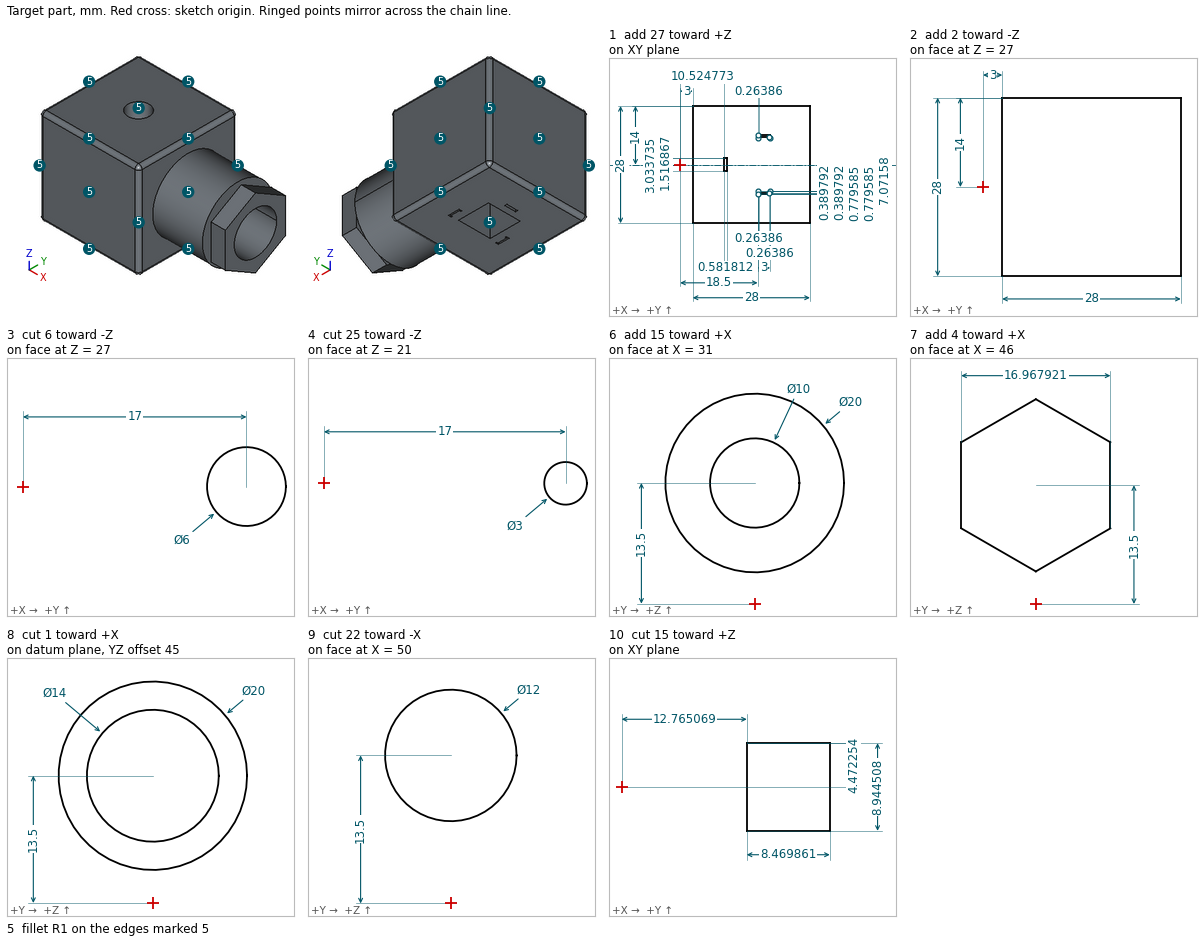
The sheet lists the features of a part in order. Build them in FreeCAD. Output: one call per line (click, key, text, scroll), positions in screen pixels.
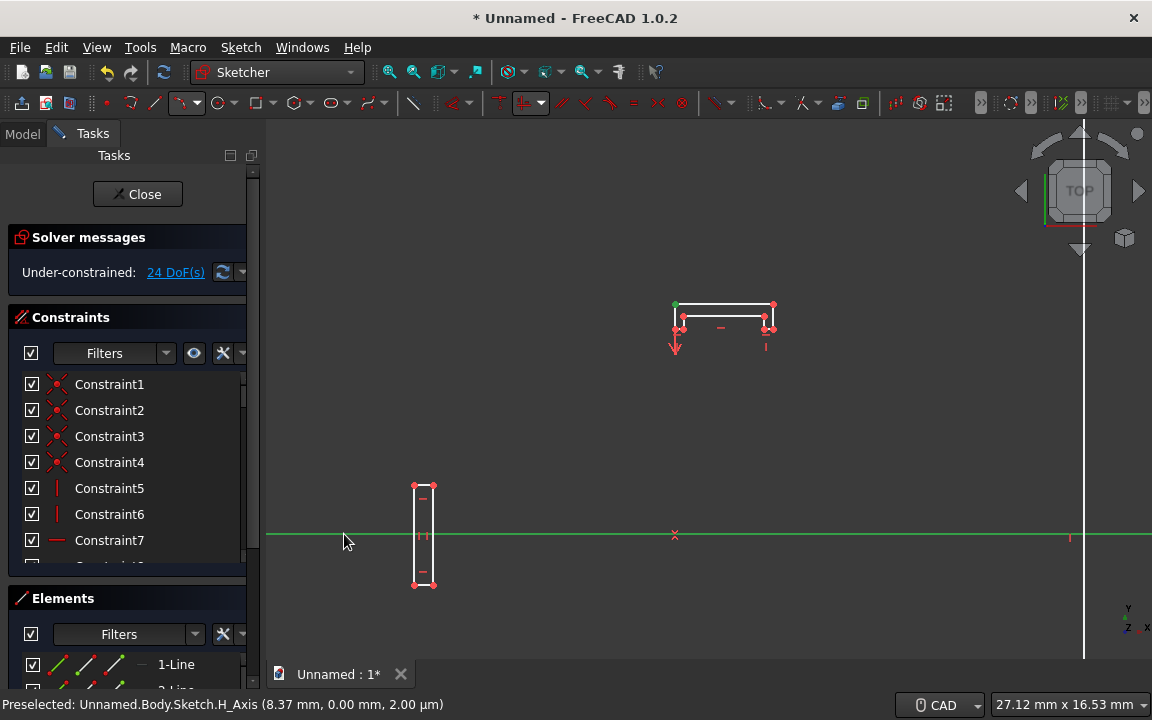
click(658, 104)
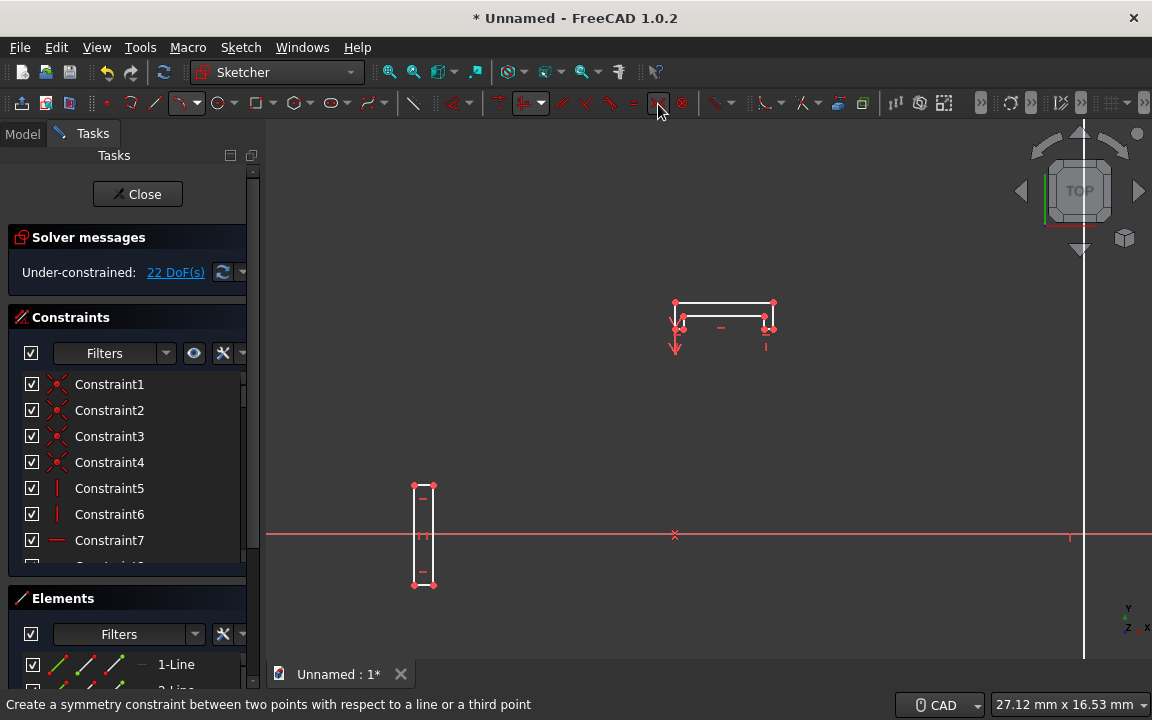
scroll(677, 304, down, 5)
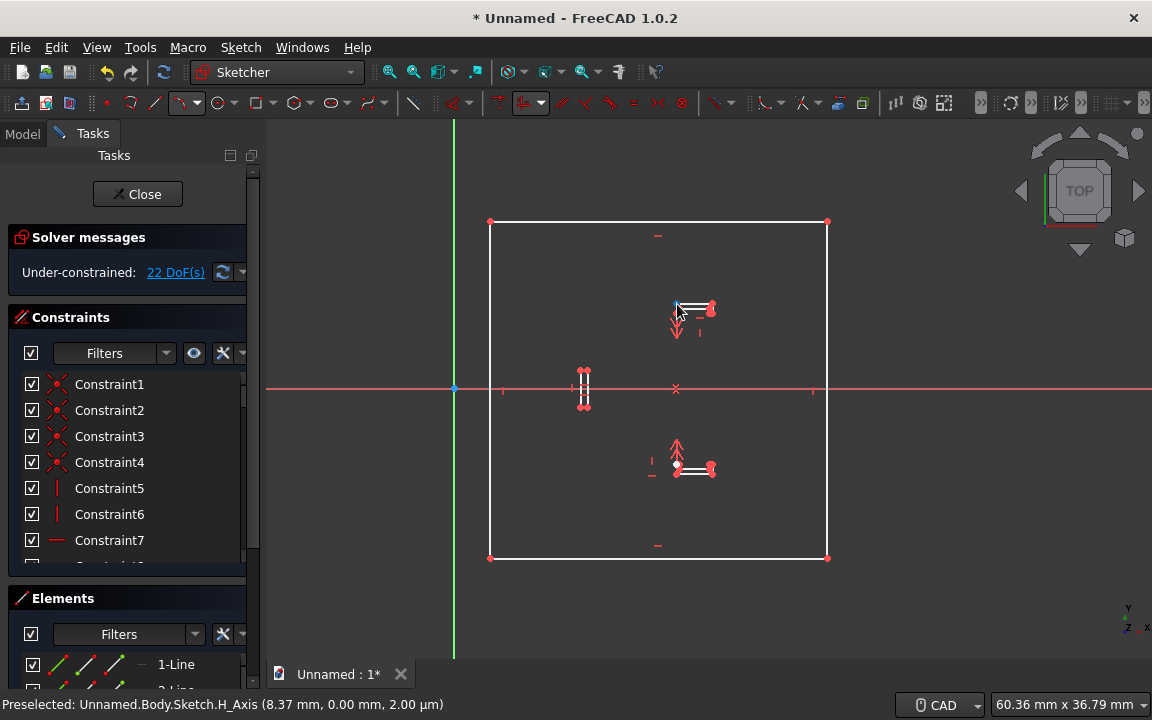
scroll(713, 465, up, 7)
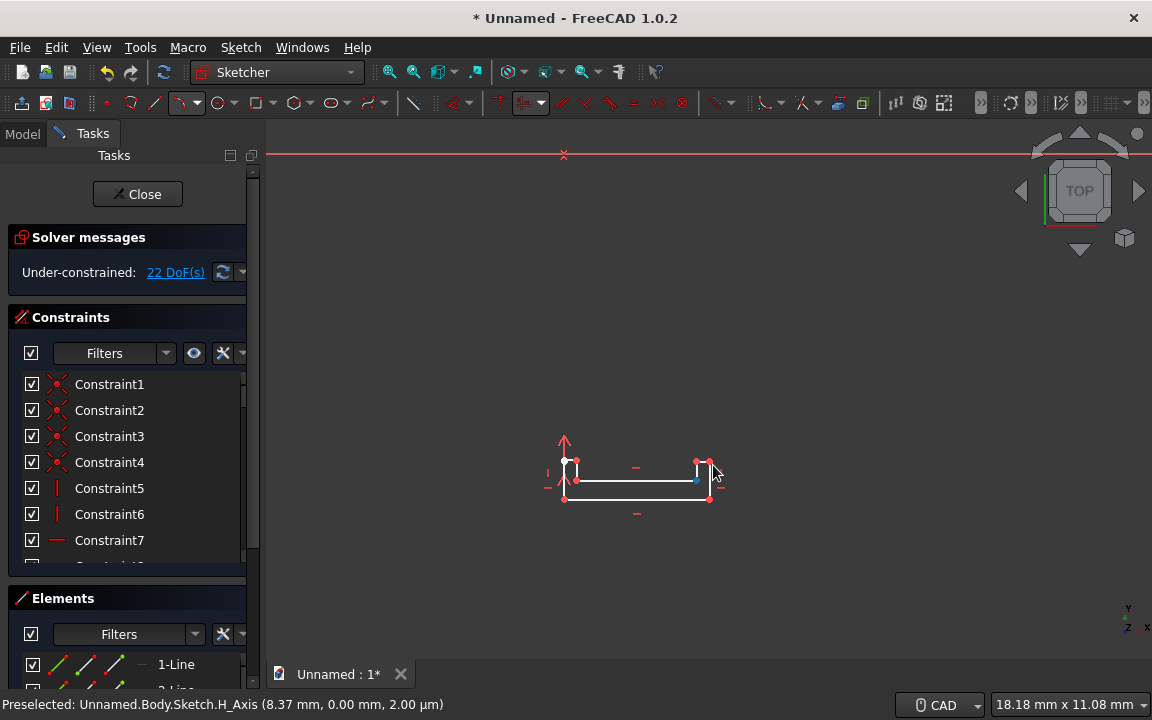
click(710, 462)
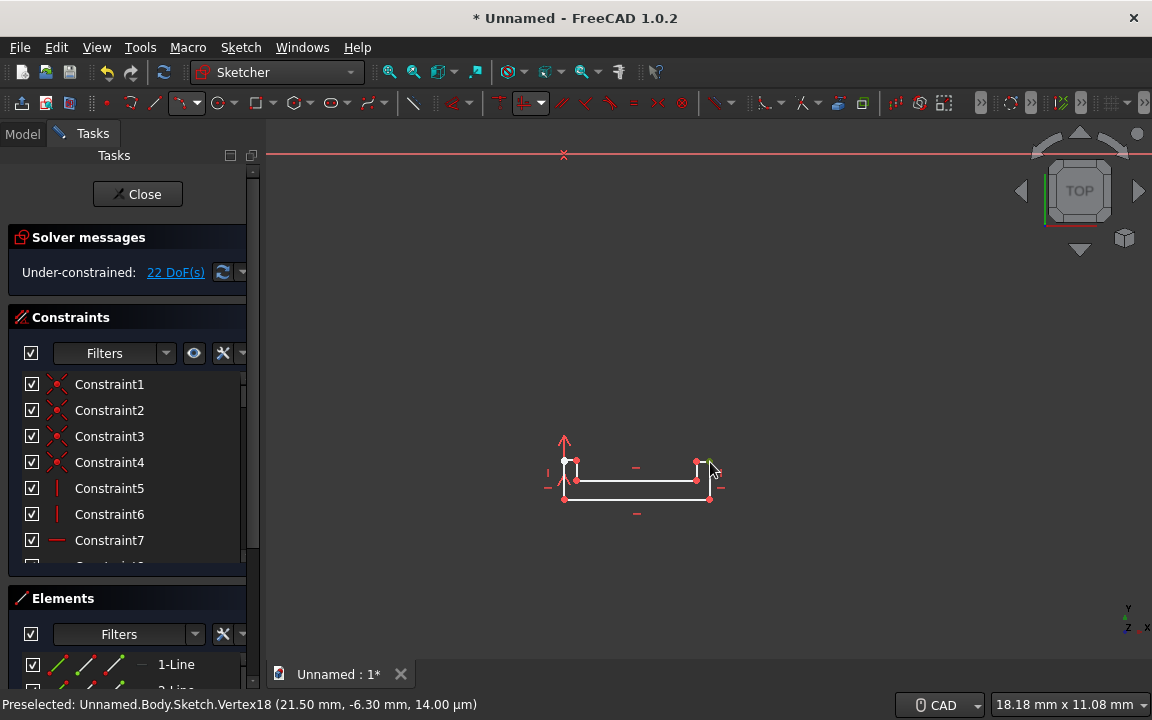
scroll(713, 466, down, 7)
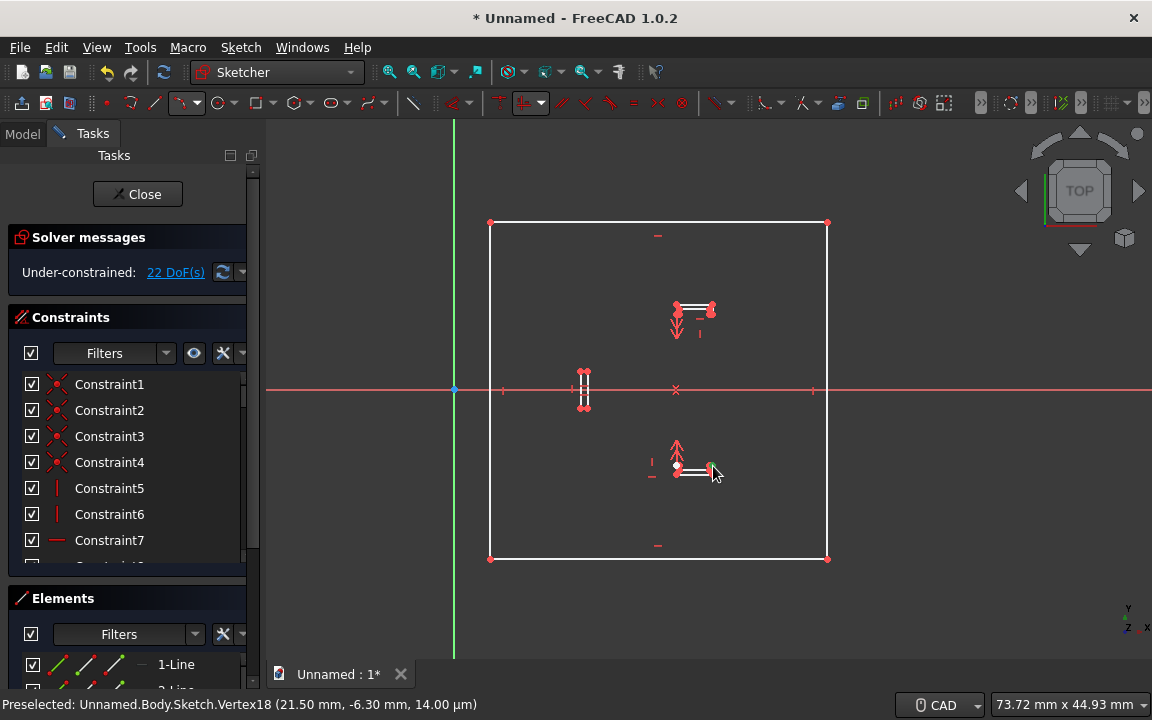
scroll(713, 314, up, 7)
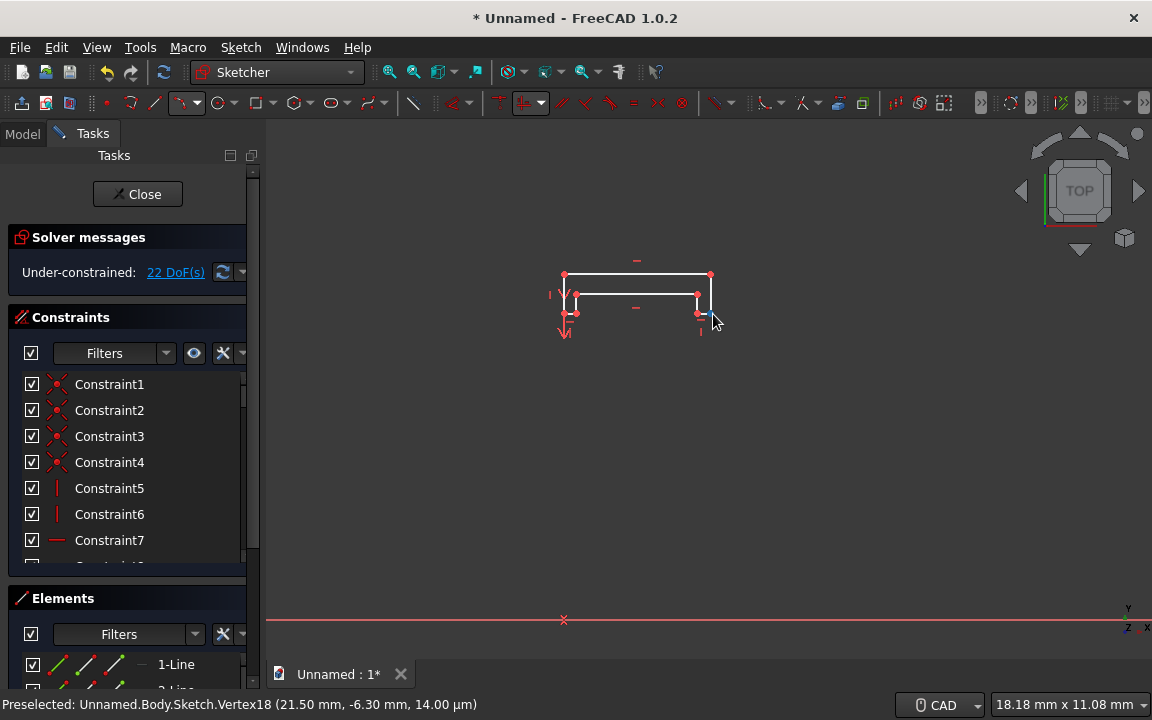
click(711, 314)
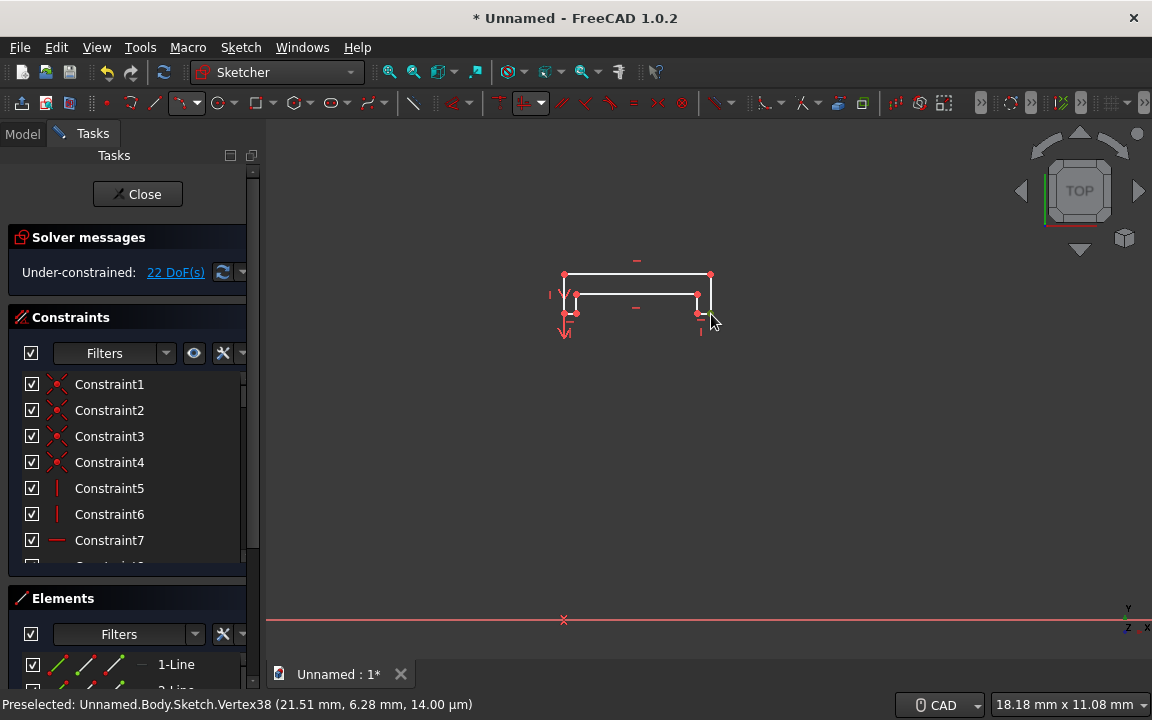
click(344, 620)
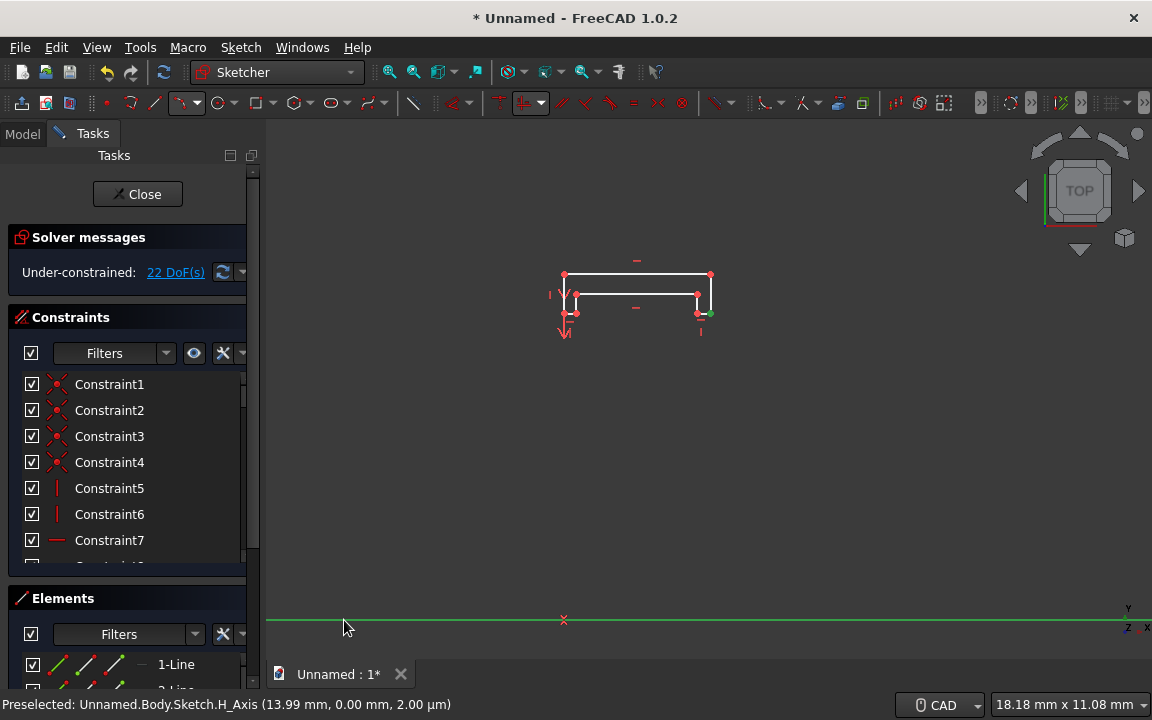
click(658, 104)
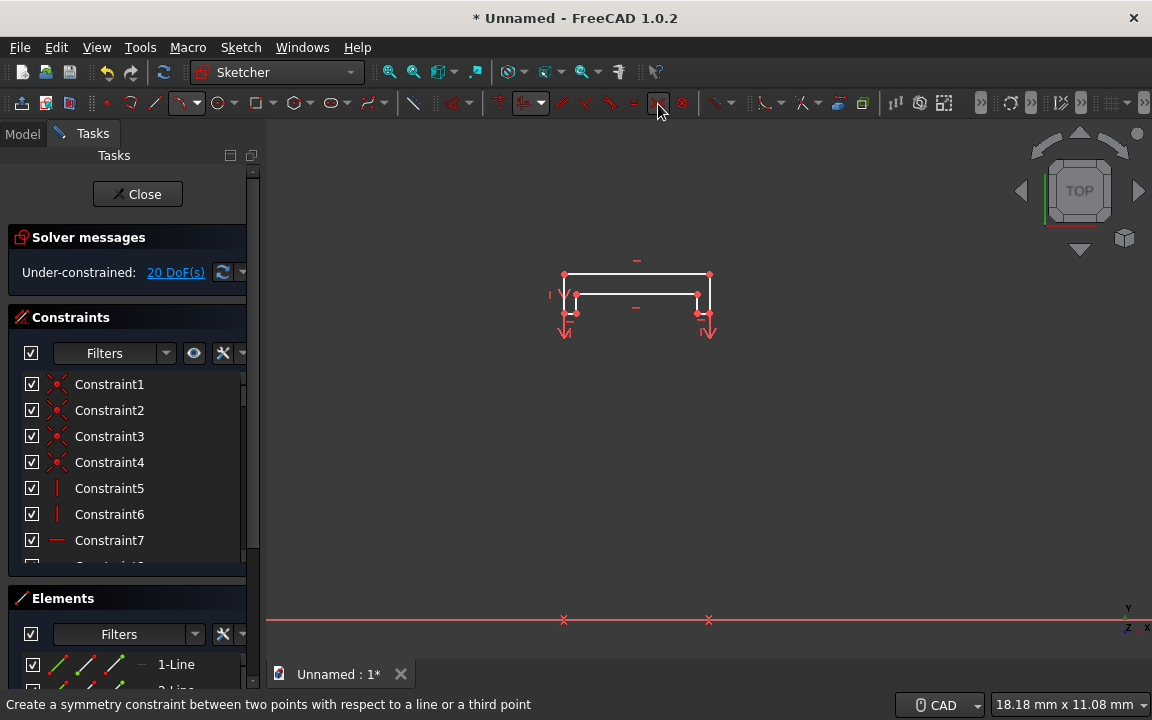
scroll(713, 313, down, 7)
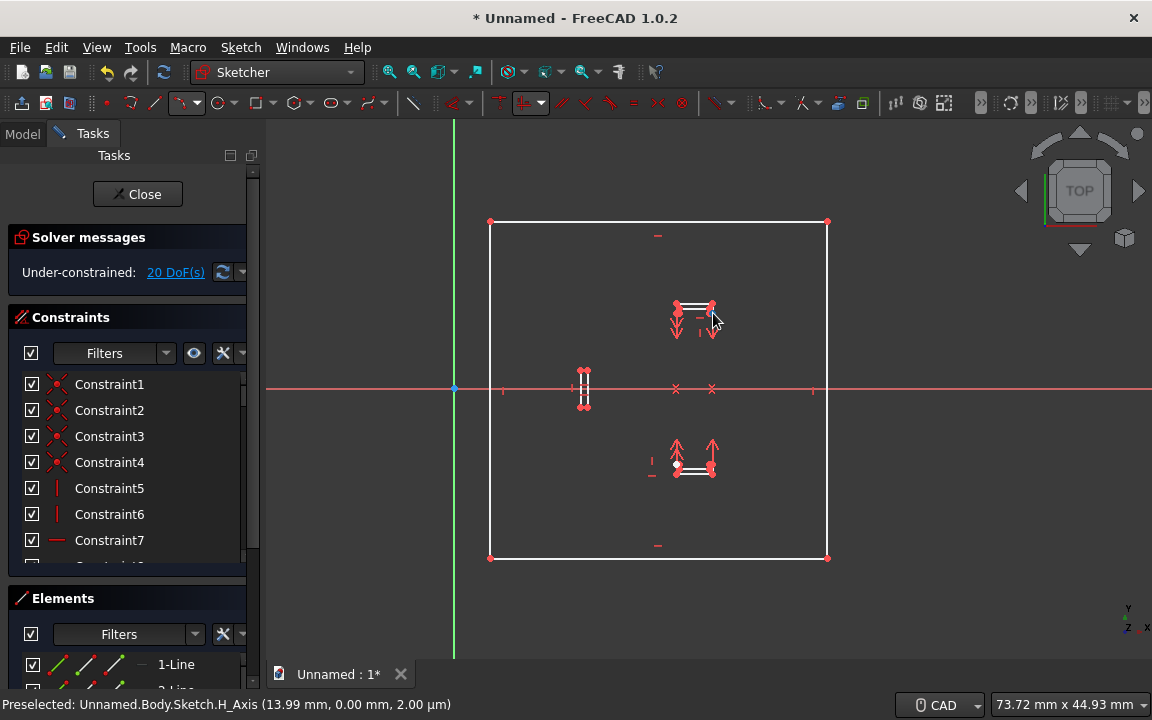
scroll(709, 469, up, 5)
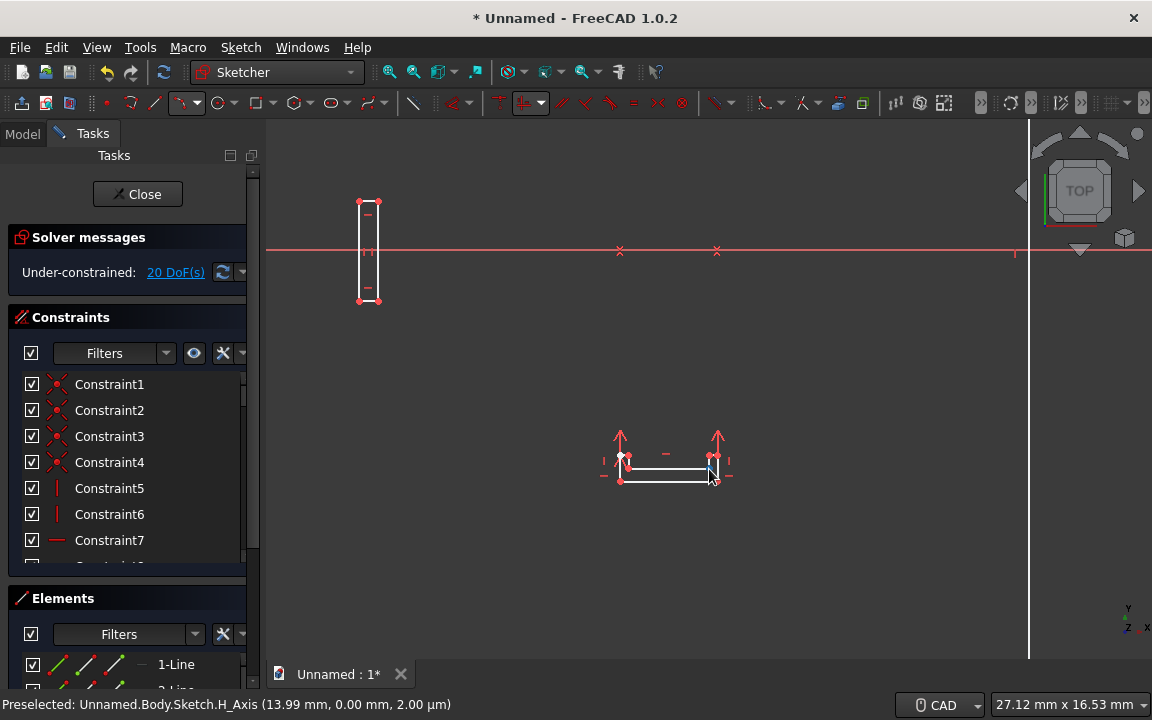
click(709, 469)